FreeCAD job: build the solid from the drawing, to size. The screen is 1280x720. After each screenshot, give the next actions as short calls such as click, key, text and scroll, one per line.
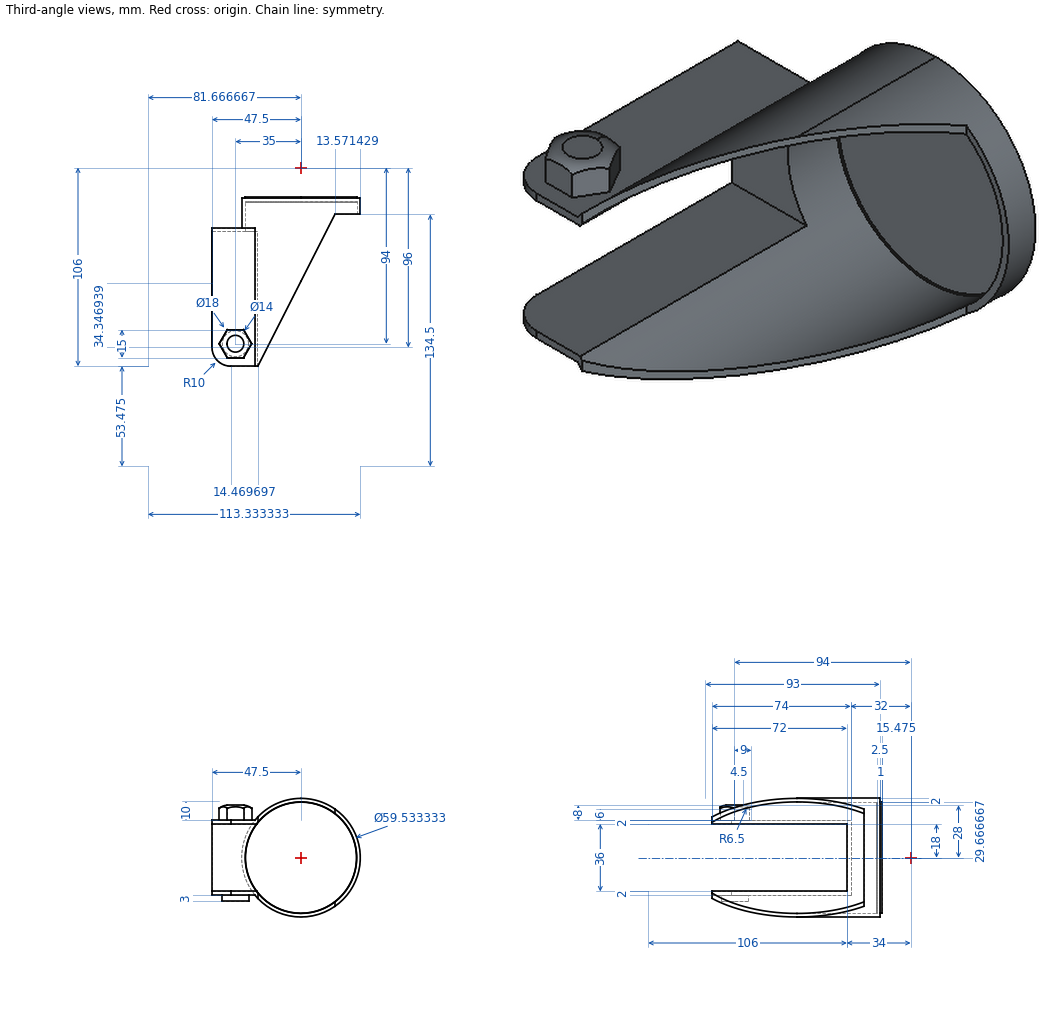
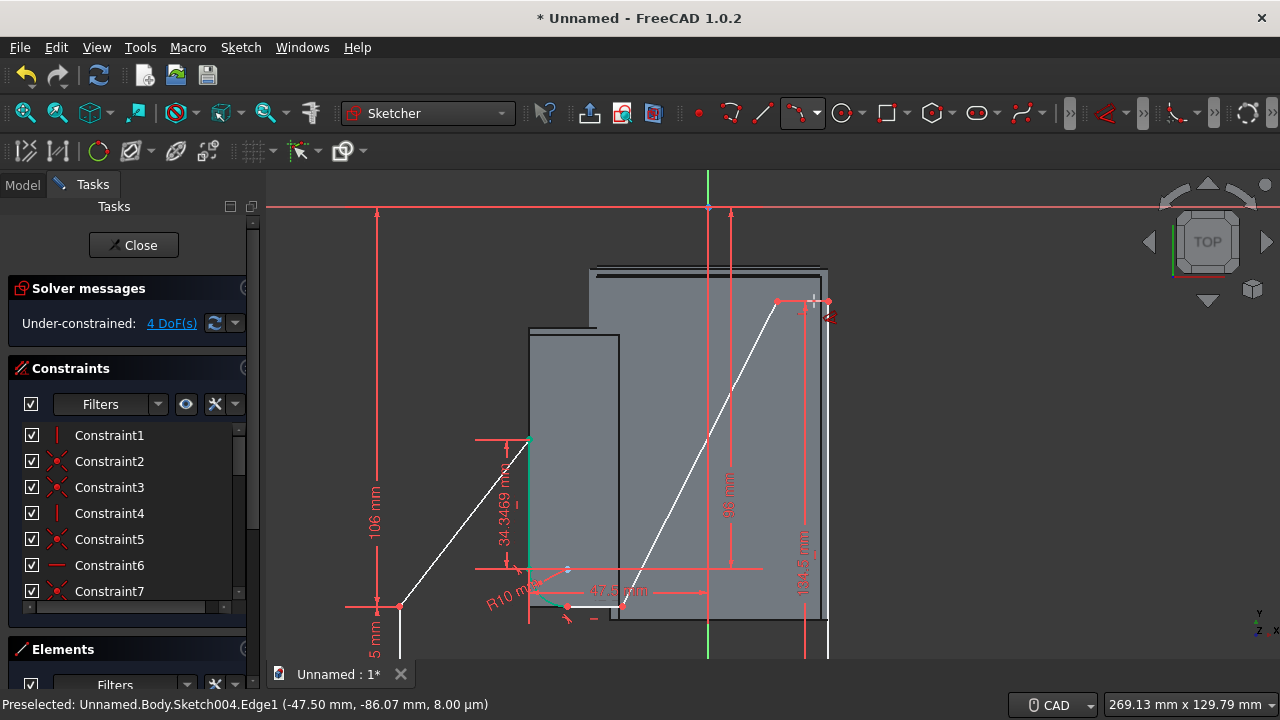
click(813, 301)
click(803, 267)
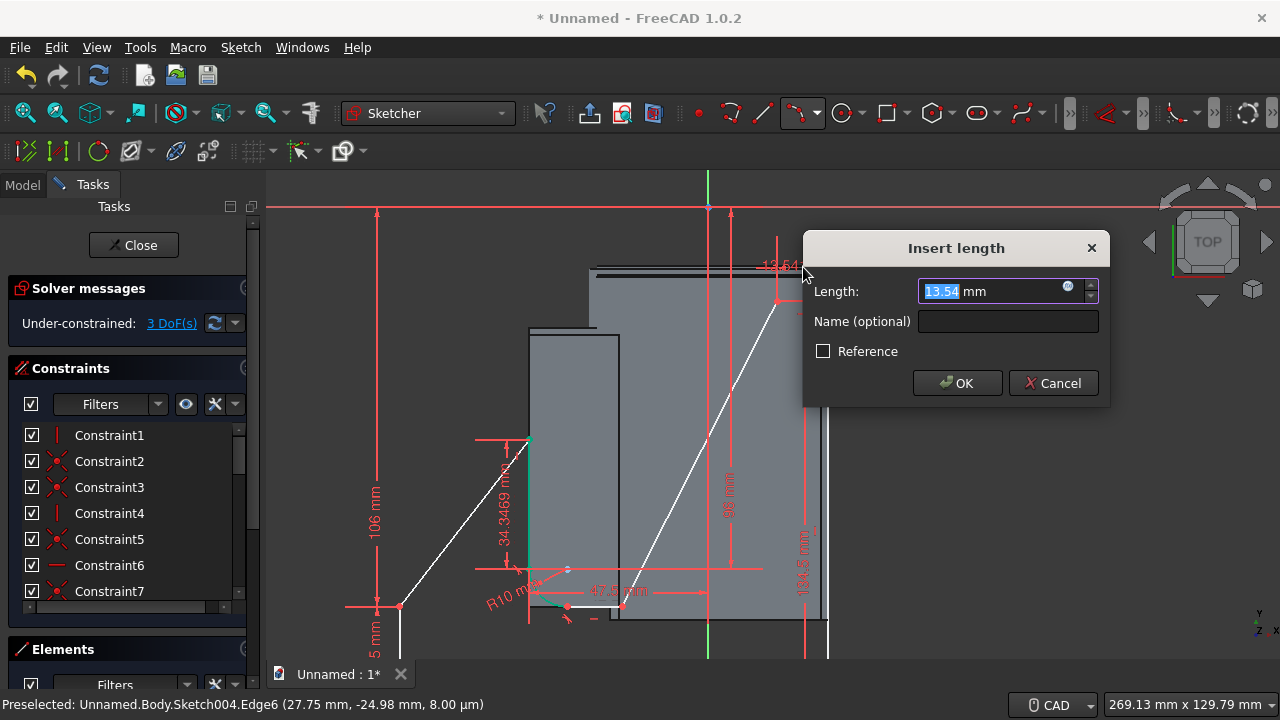
text(13.571429)
key(Return)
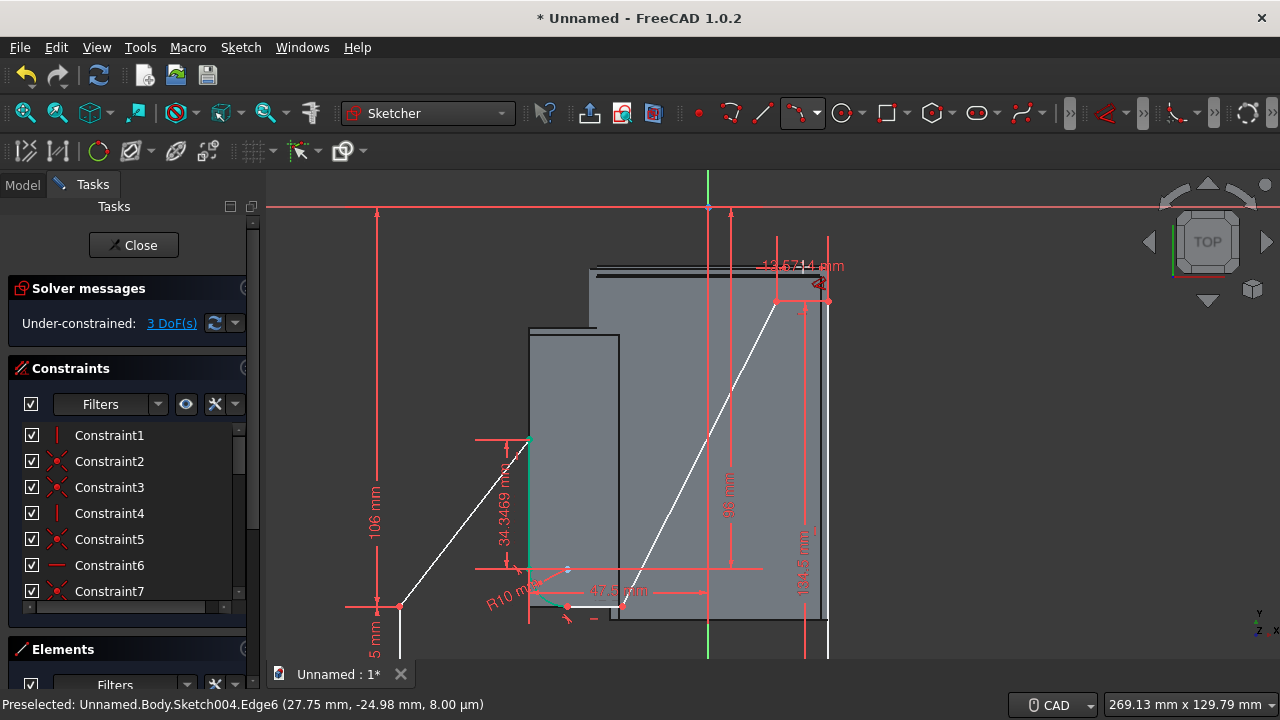
click(606, 607)
click(595, 549)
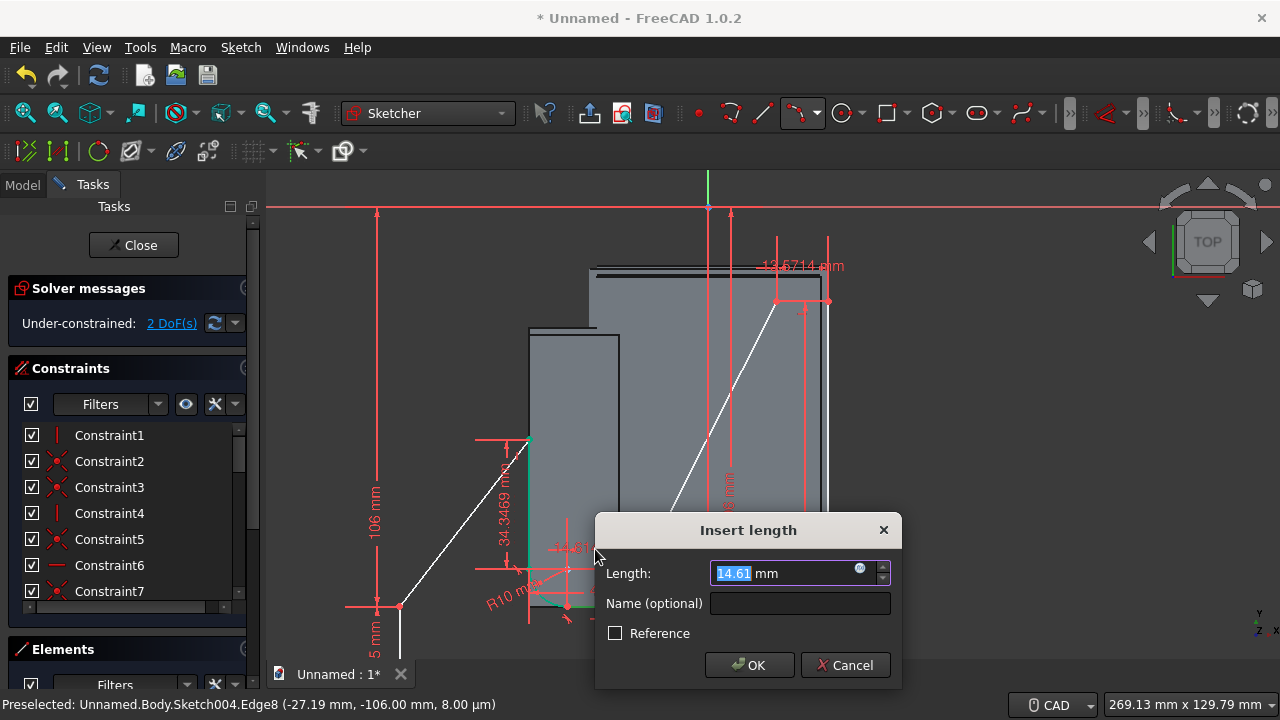
text(14.469697)
key(Return)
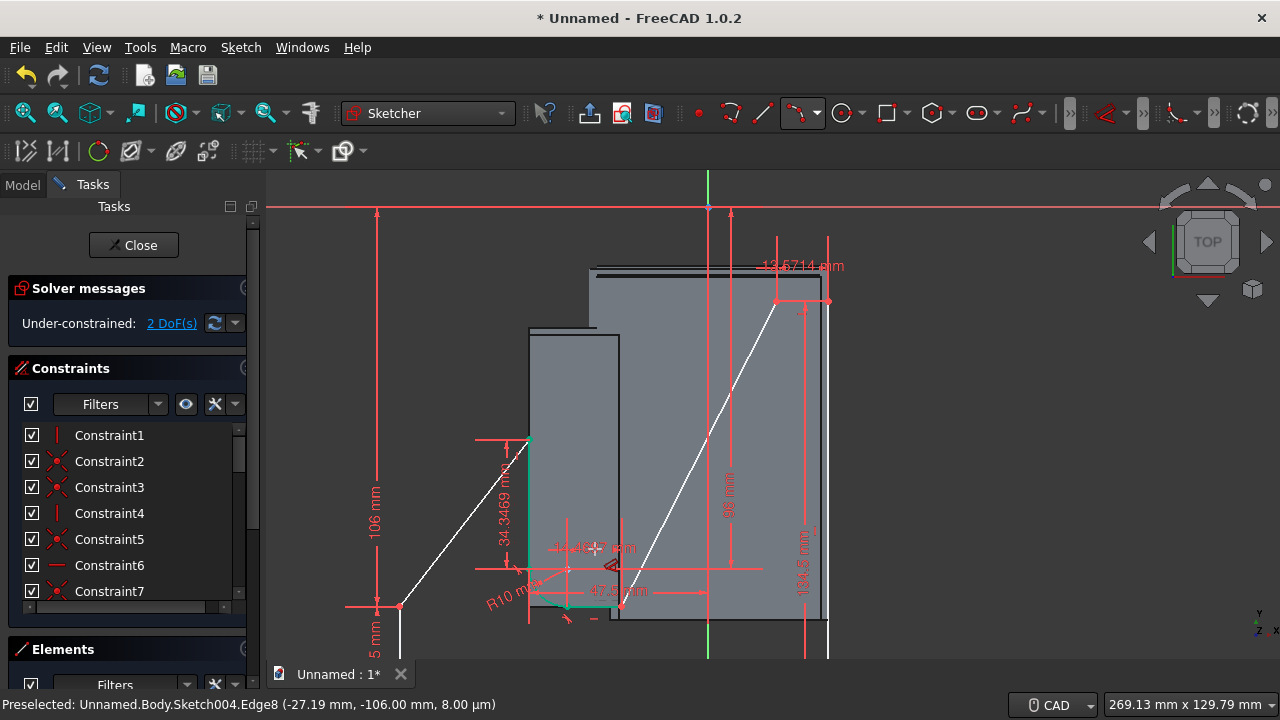
scroll(814, 301, down, 3)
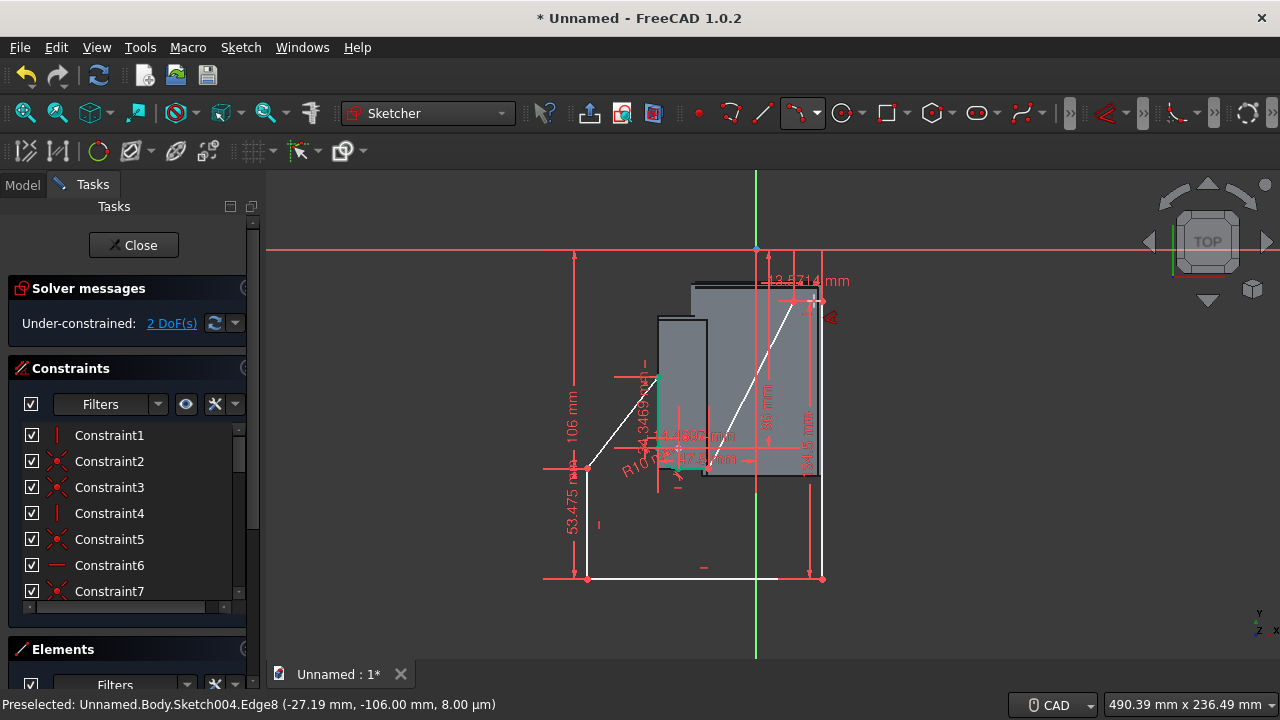
click(657, 579)
click(704, 613)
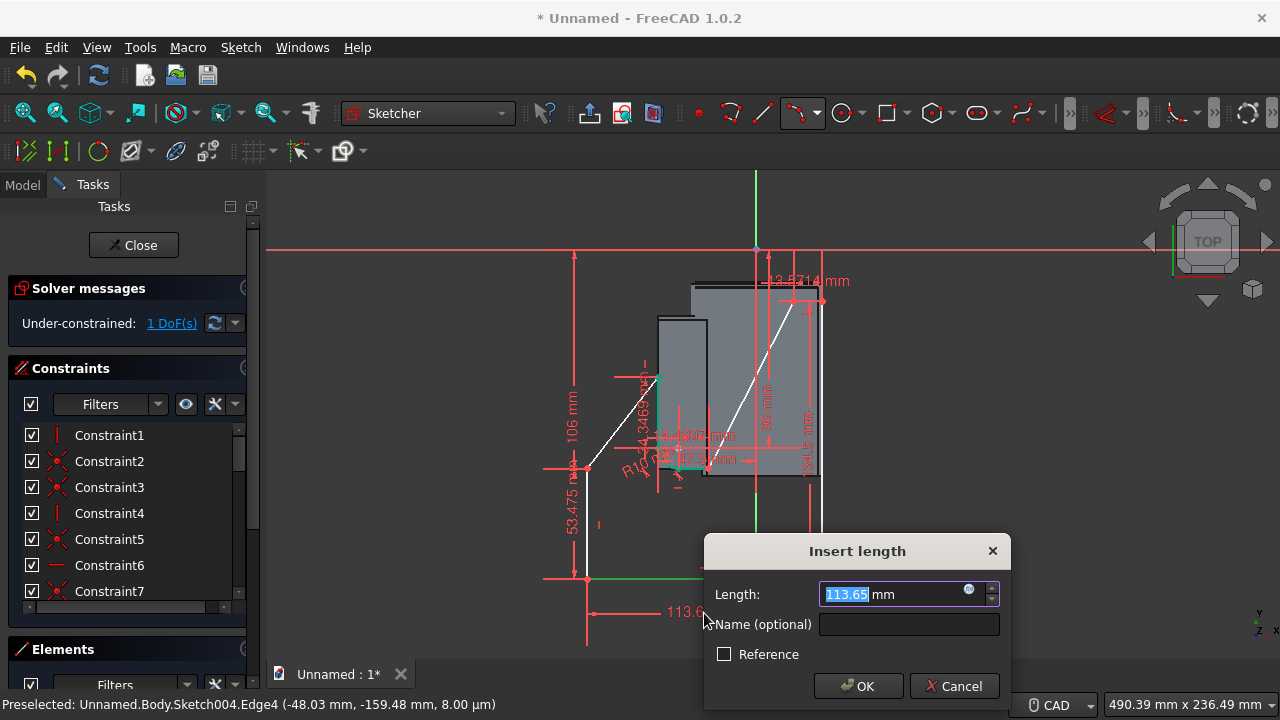
text(113.333333)
key(Return)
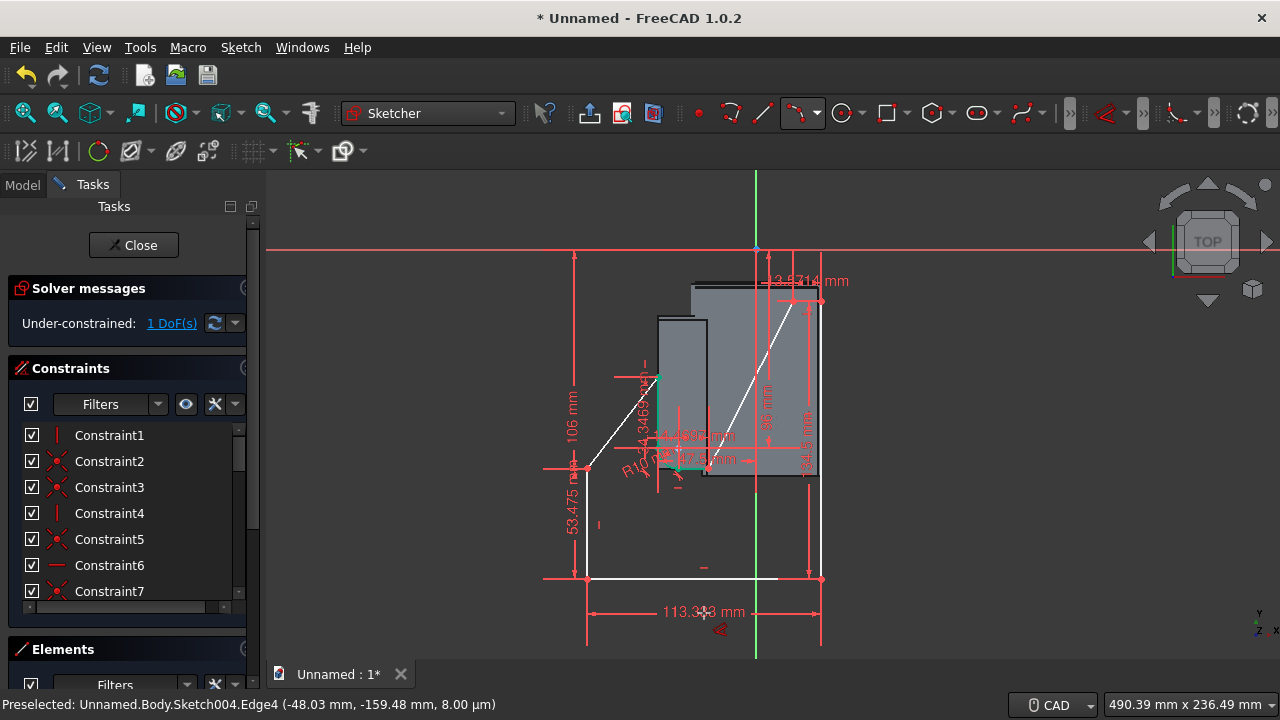
click(587, 469)
click(672, 216)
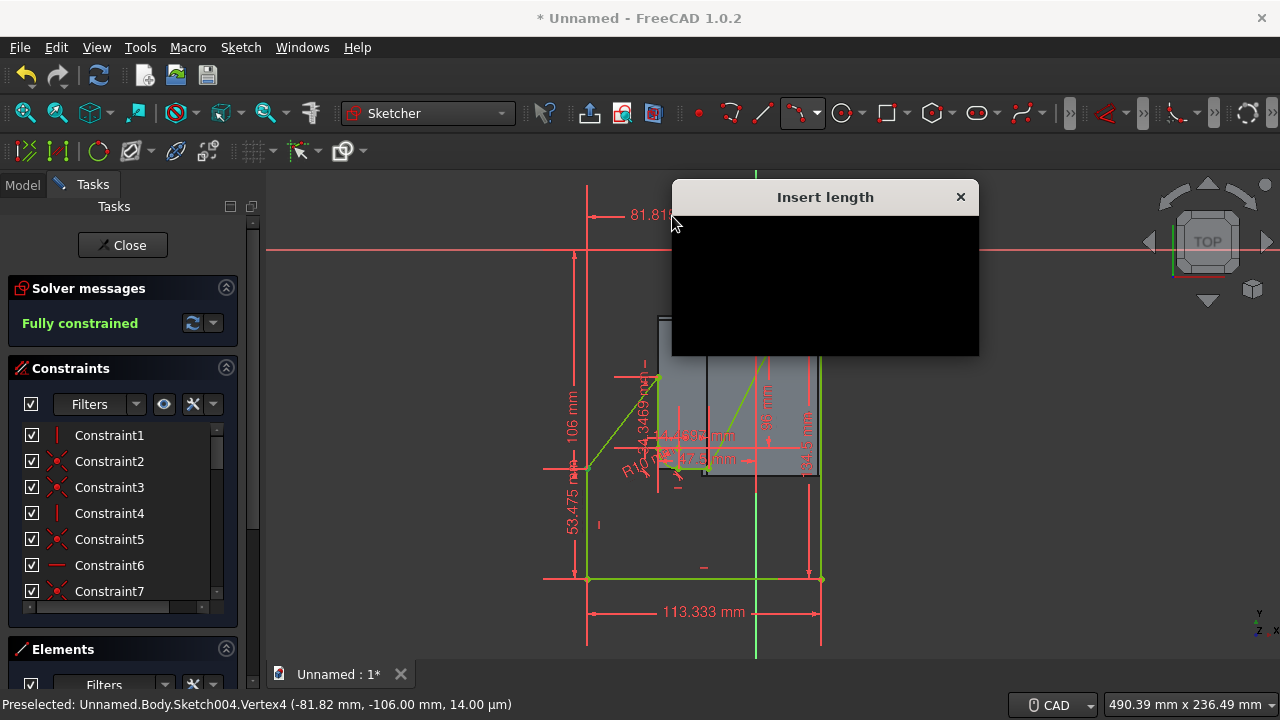
text(81.666667)
key(Return)
key(Escape)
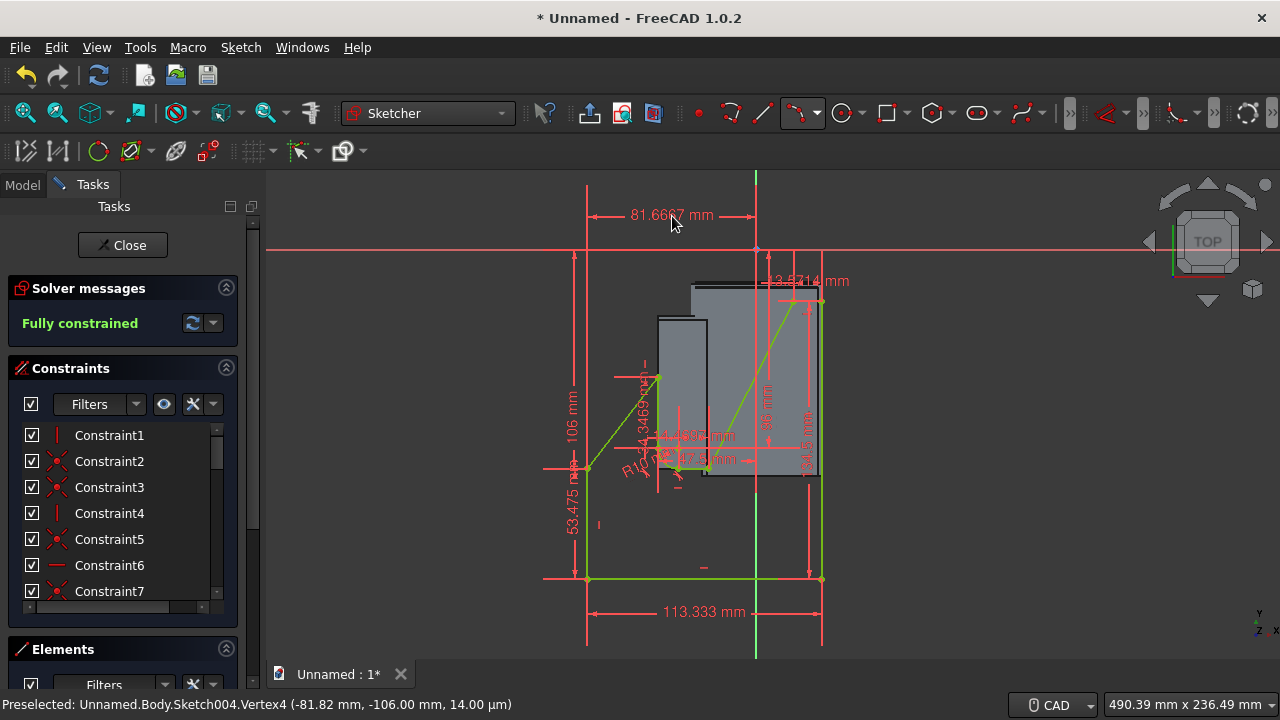
click(123, 245)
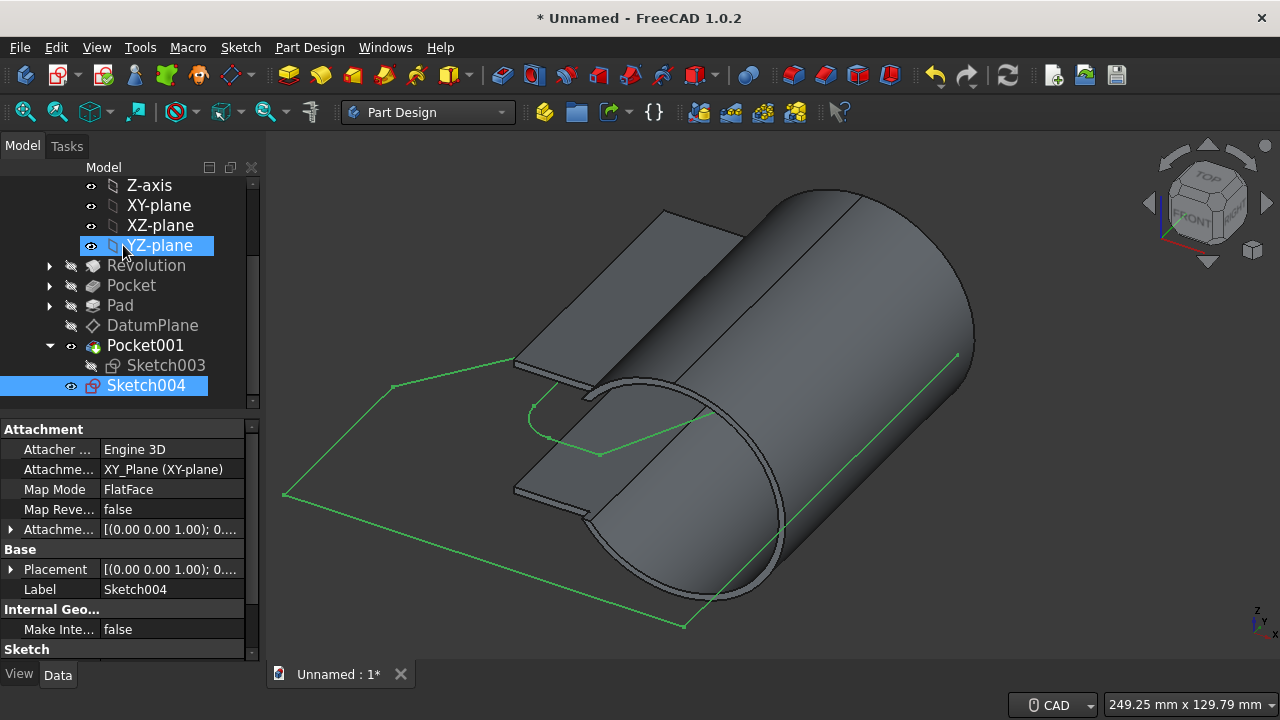
click(504, 76)